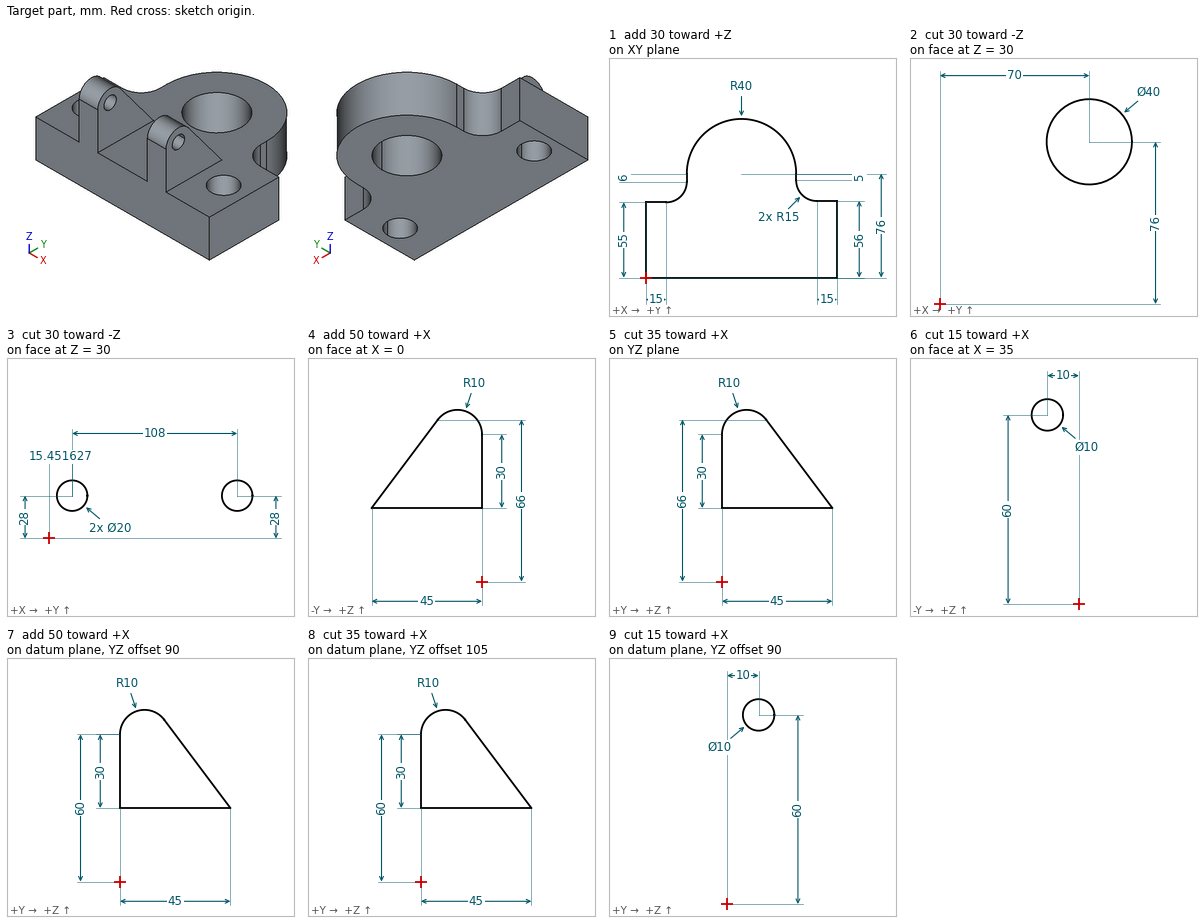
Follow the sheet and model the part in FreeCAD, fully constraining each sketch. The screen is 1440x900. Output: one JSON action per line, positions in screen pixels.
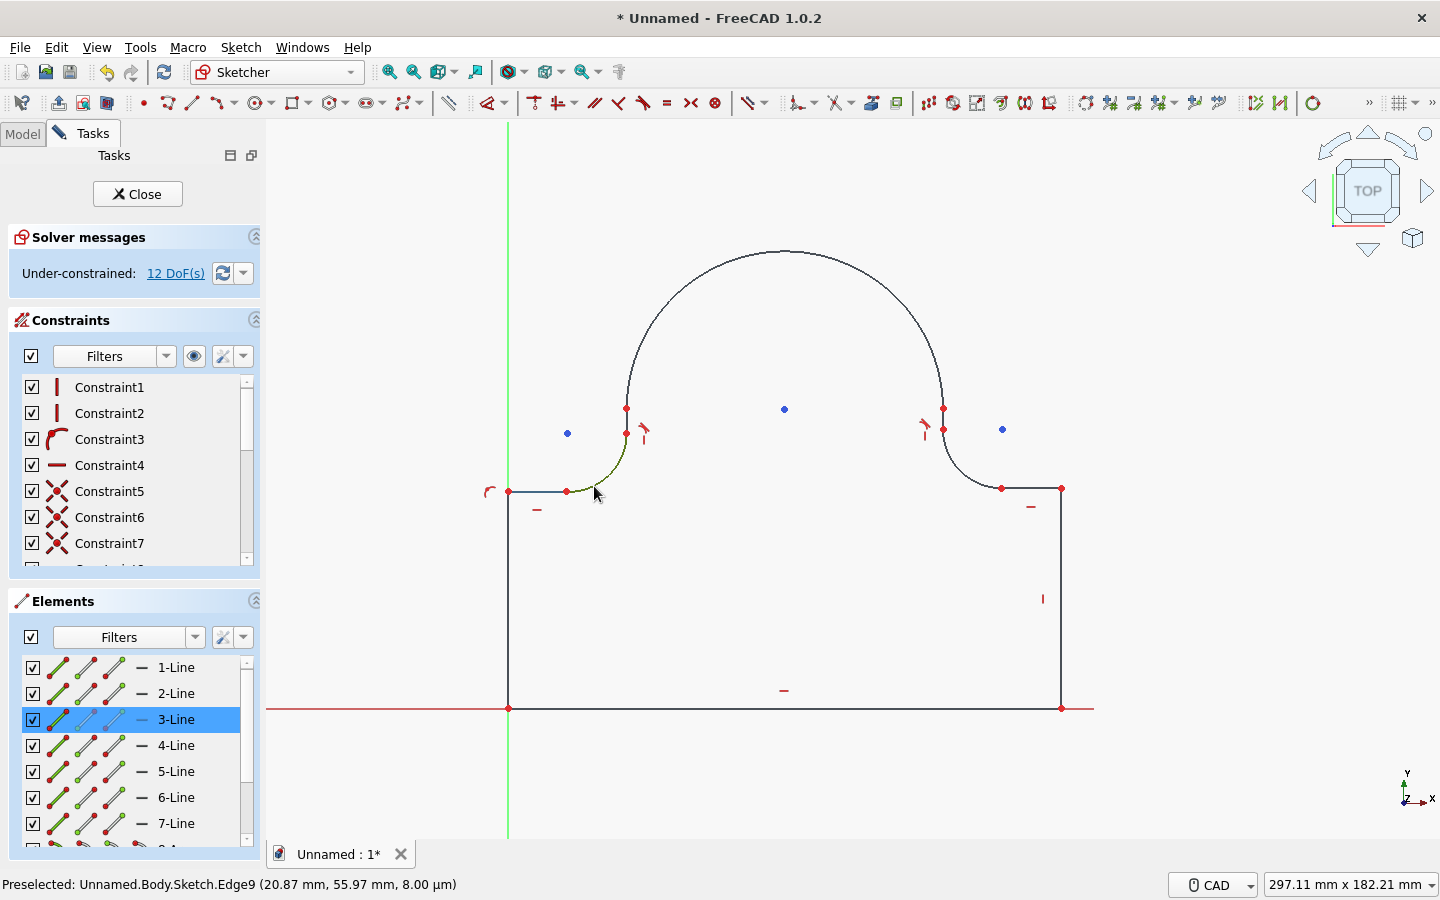
{"action": "key", "text": "t"}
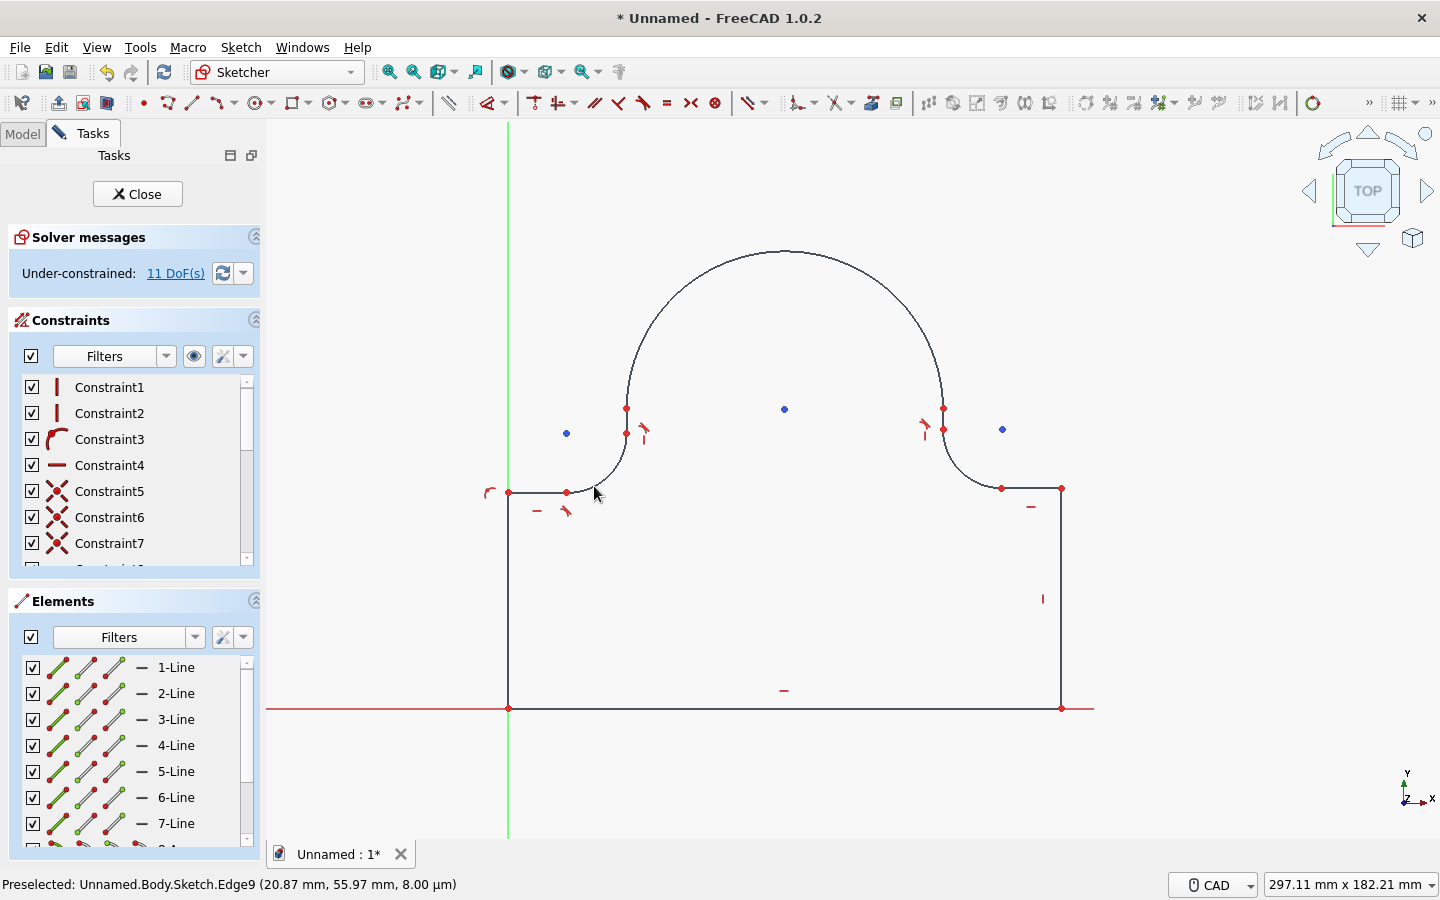
{"action": "left_click", "coordinate": [1044, 488]}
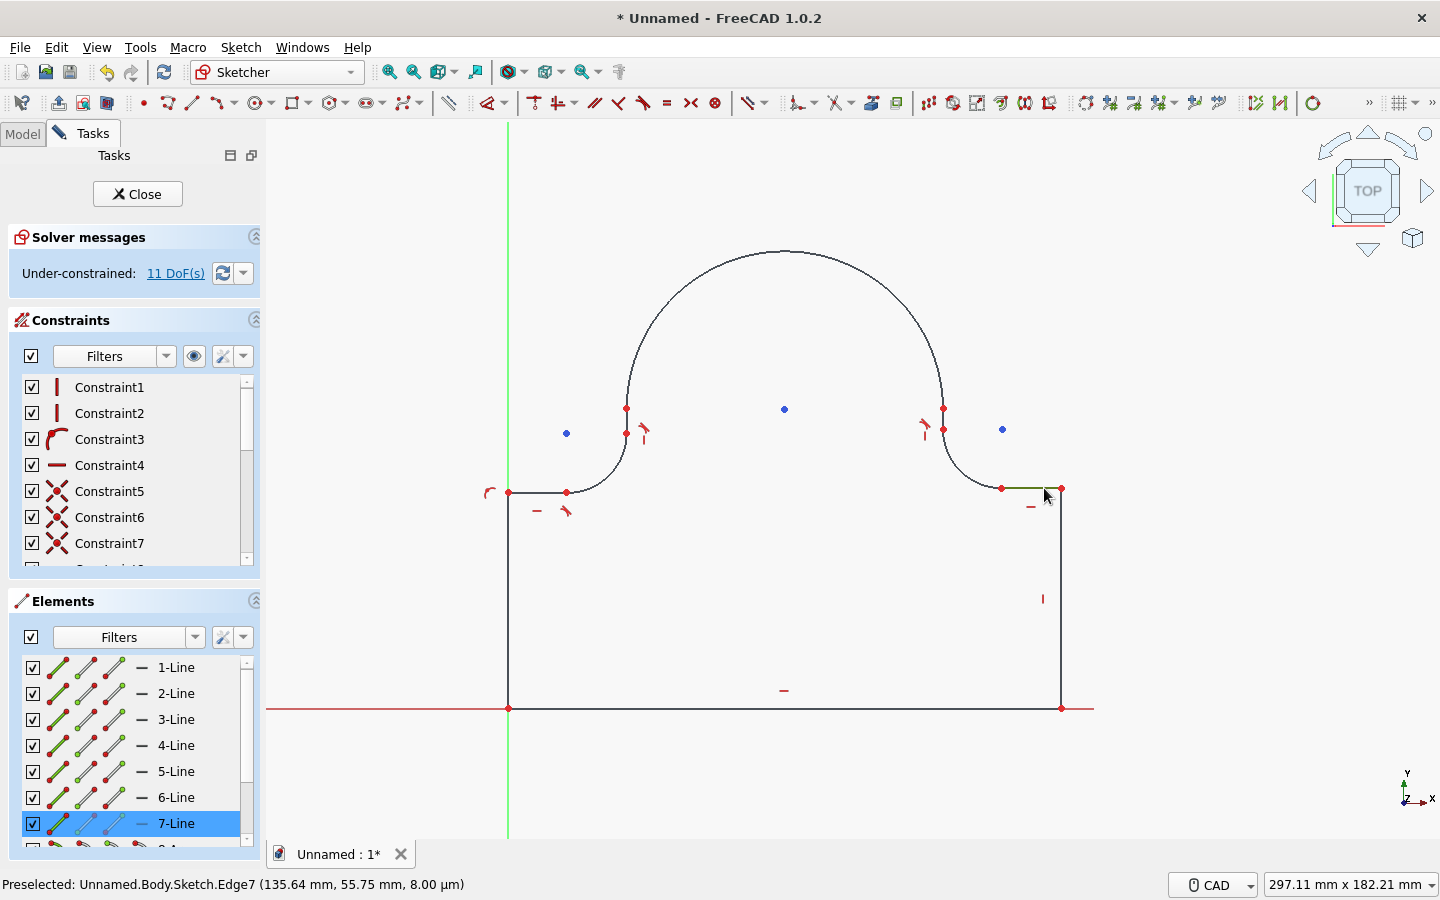
{"action": "left_click", "coordinate": [949, 456]}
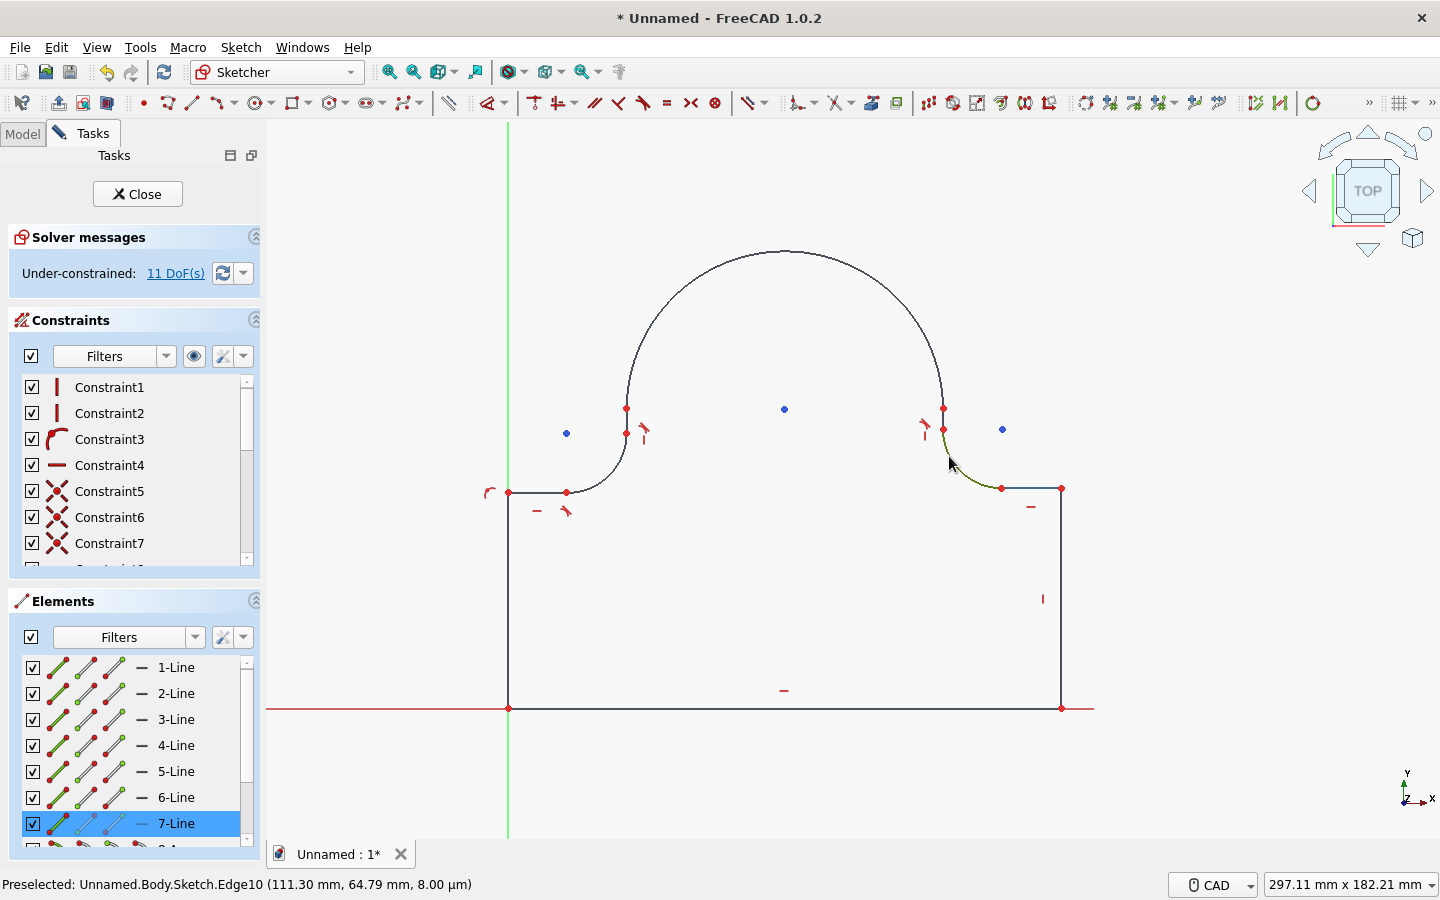
{"action": "left_click", "coordinate": [644, 104]}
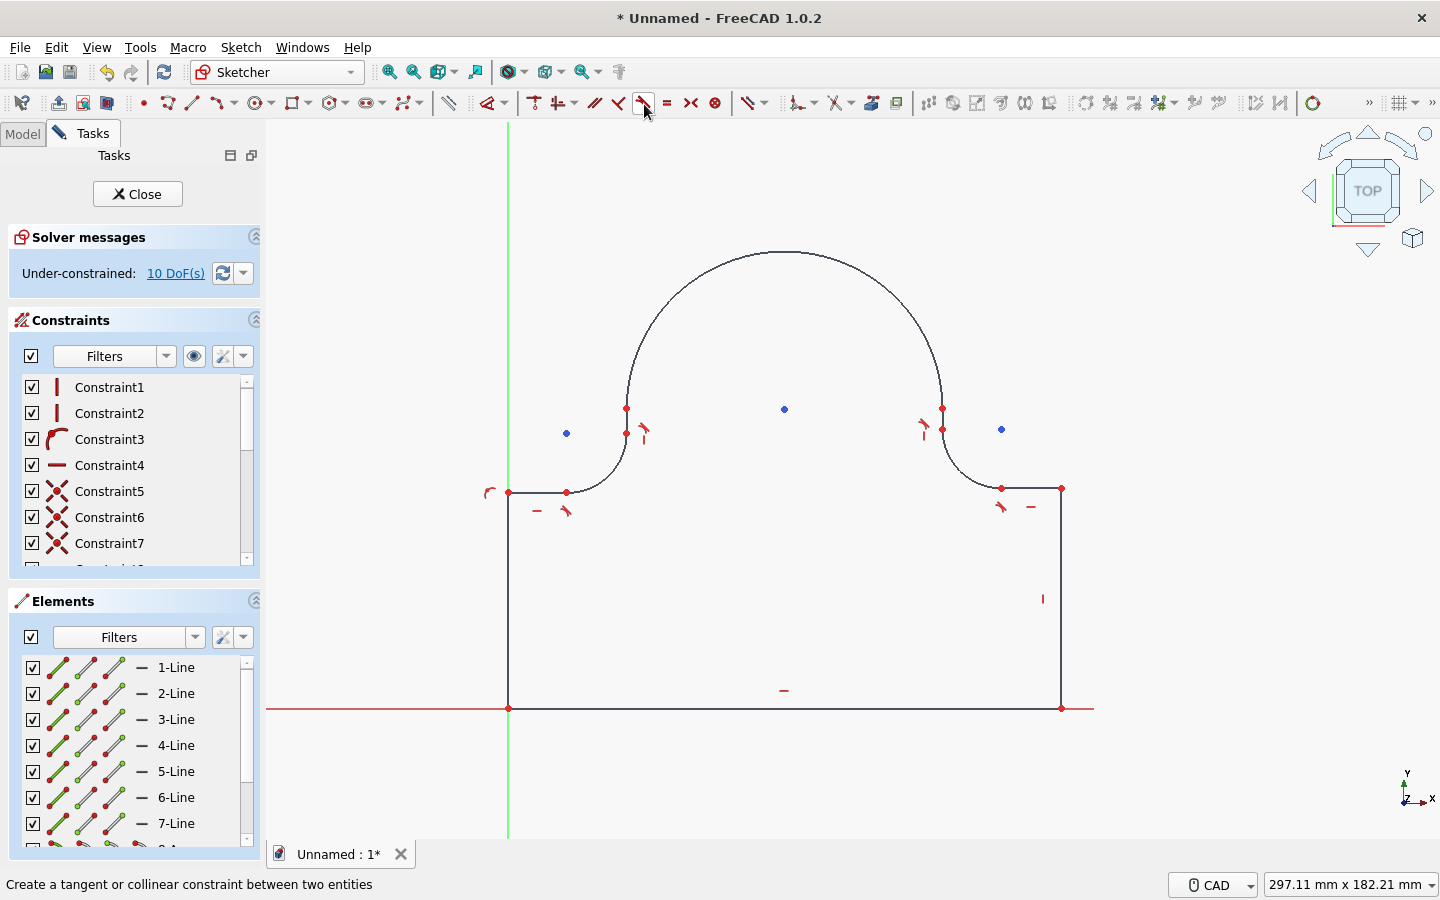
{"action": "left_click", "coordinate": [594, 486]}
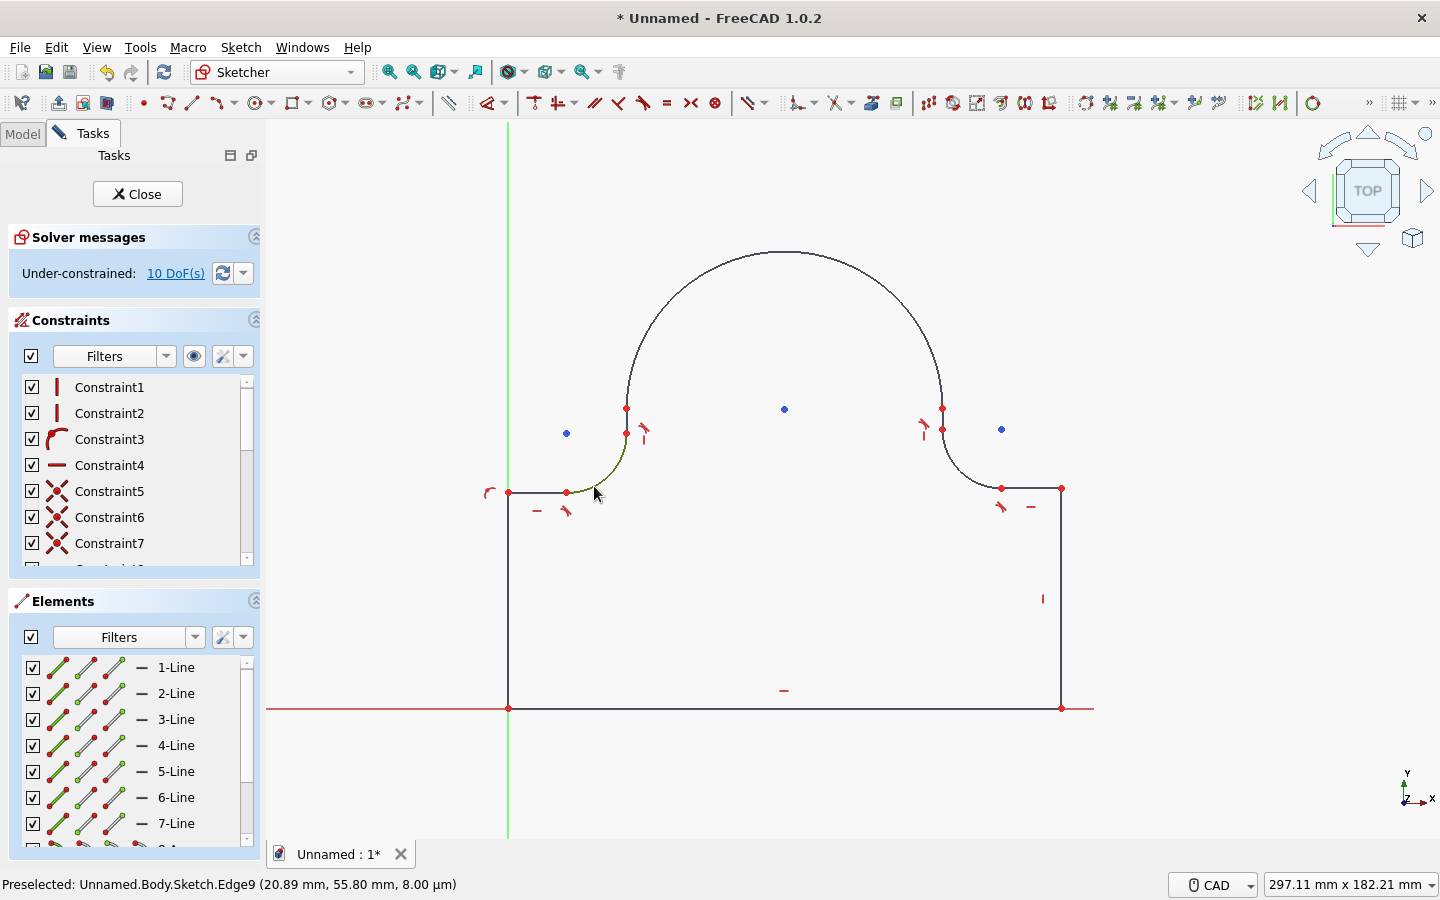
{"action": "left_click", "coordinate": [949, 456]}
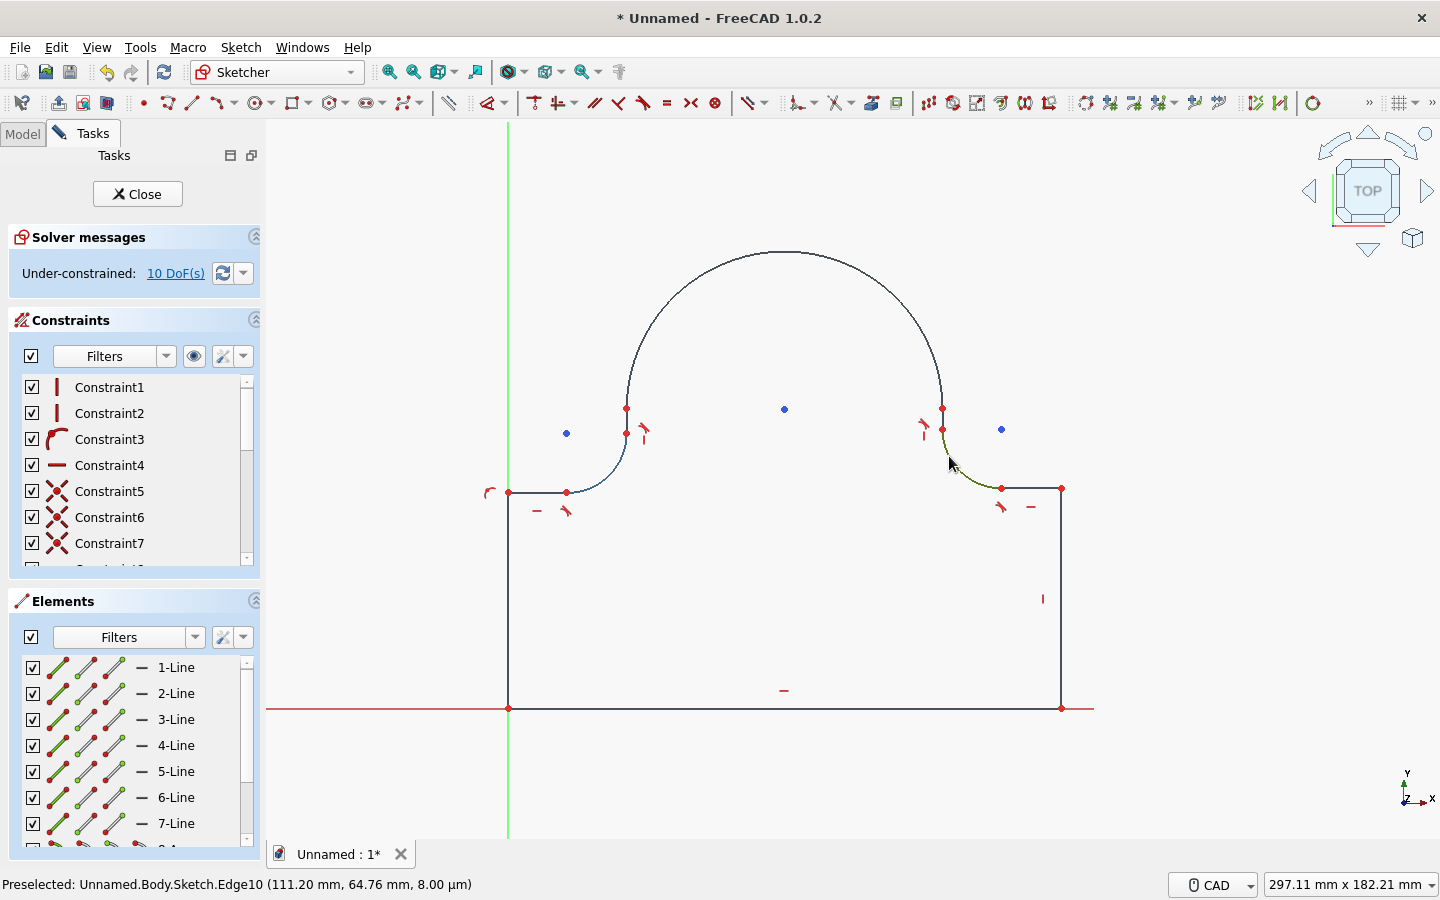
{"action": "left_click", "coordinate": [668, 104]}